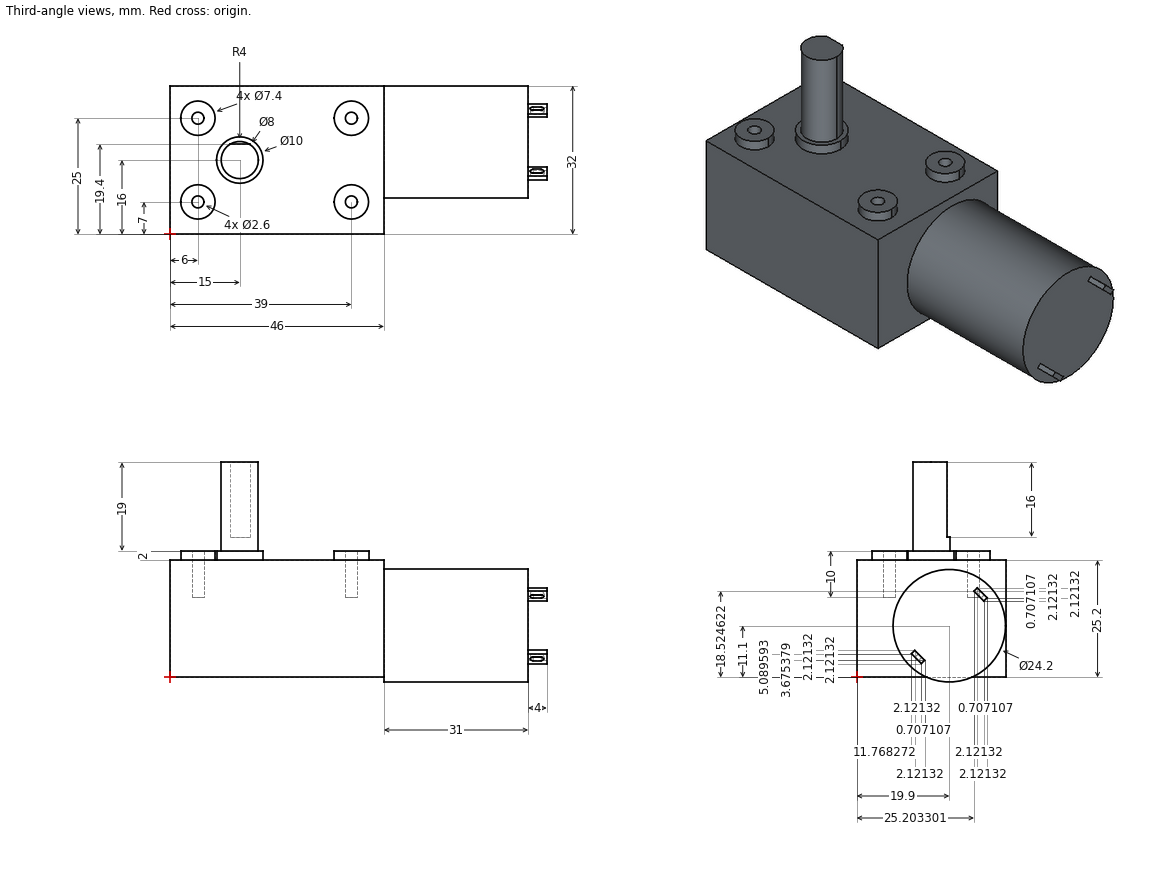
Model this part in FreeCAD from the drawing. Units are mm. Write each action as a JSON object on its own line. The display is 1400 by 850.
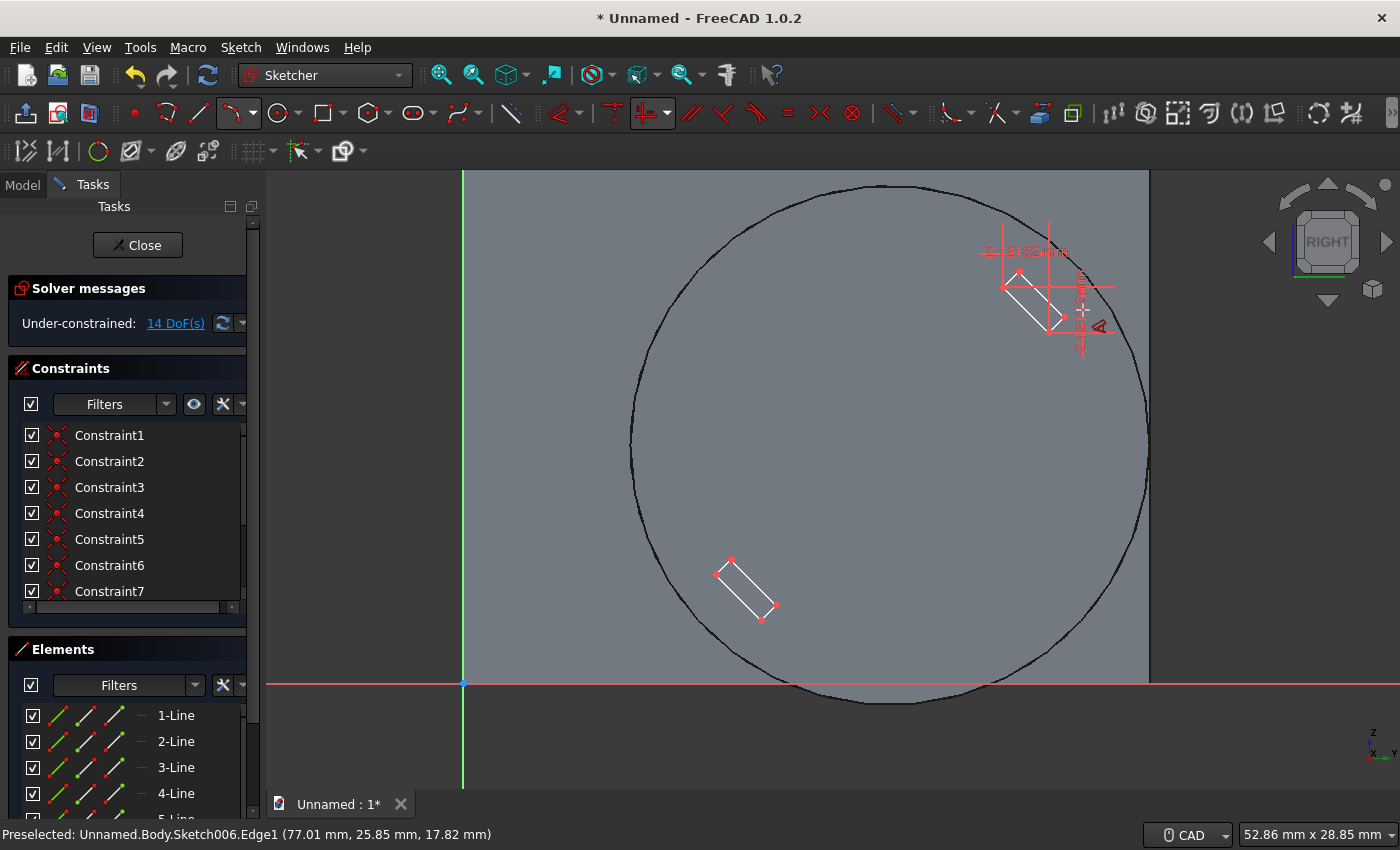
{"action": "left_click", "coordinate": [1050, 304]}
{"action": "left_click", "coordinate": [1041, 352]}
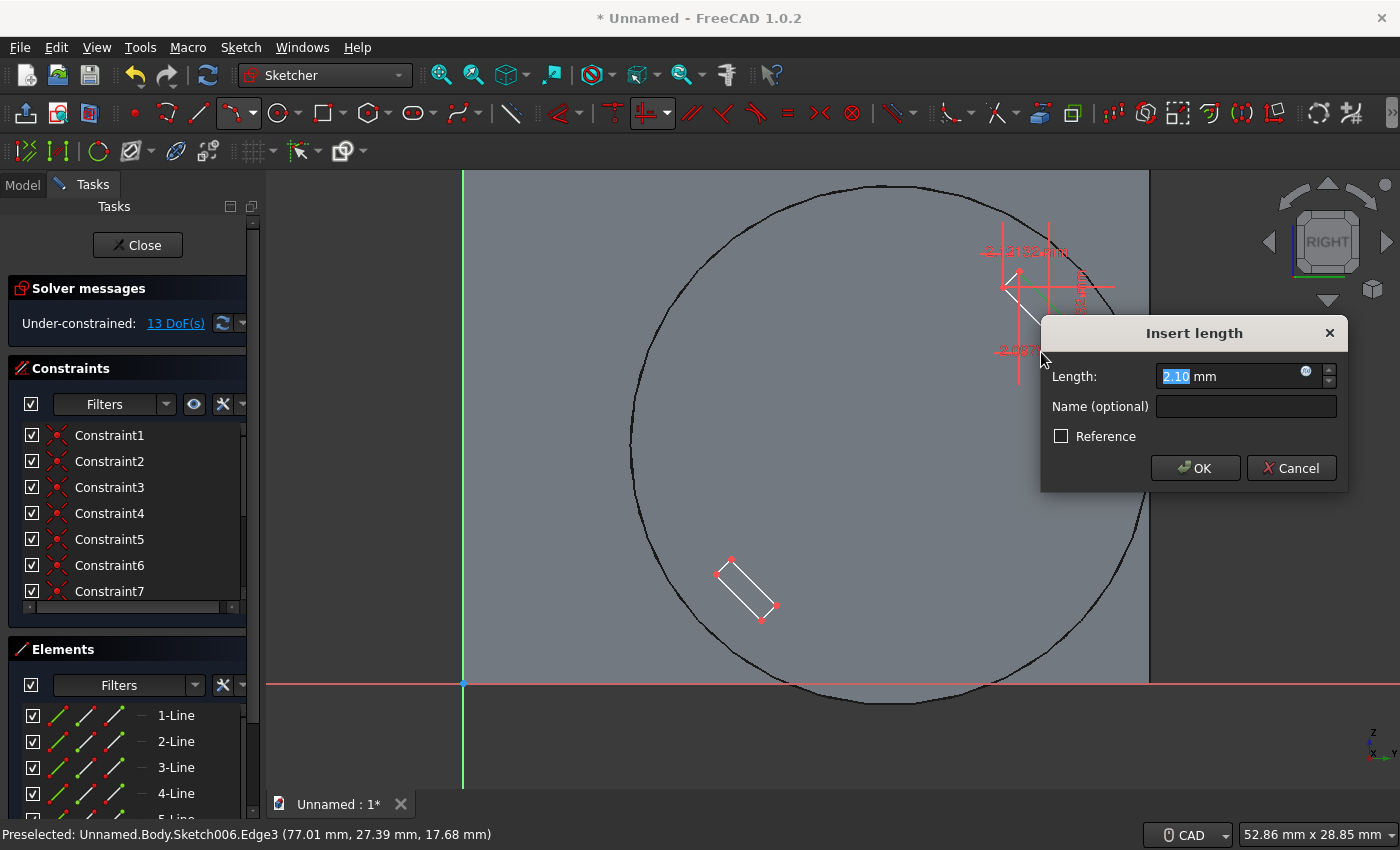
{"action": "type", "text": "2.12132"}
{"action": "key", "text": "Return"}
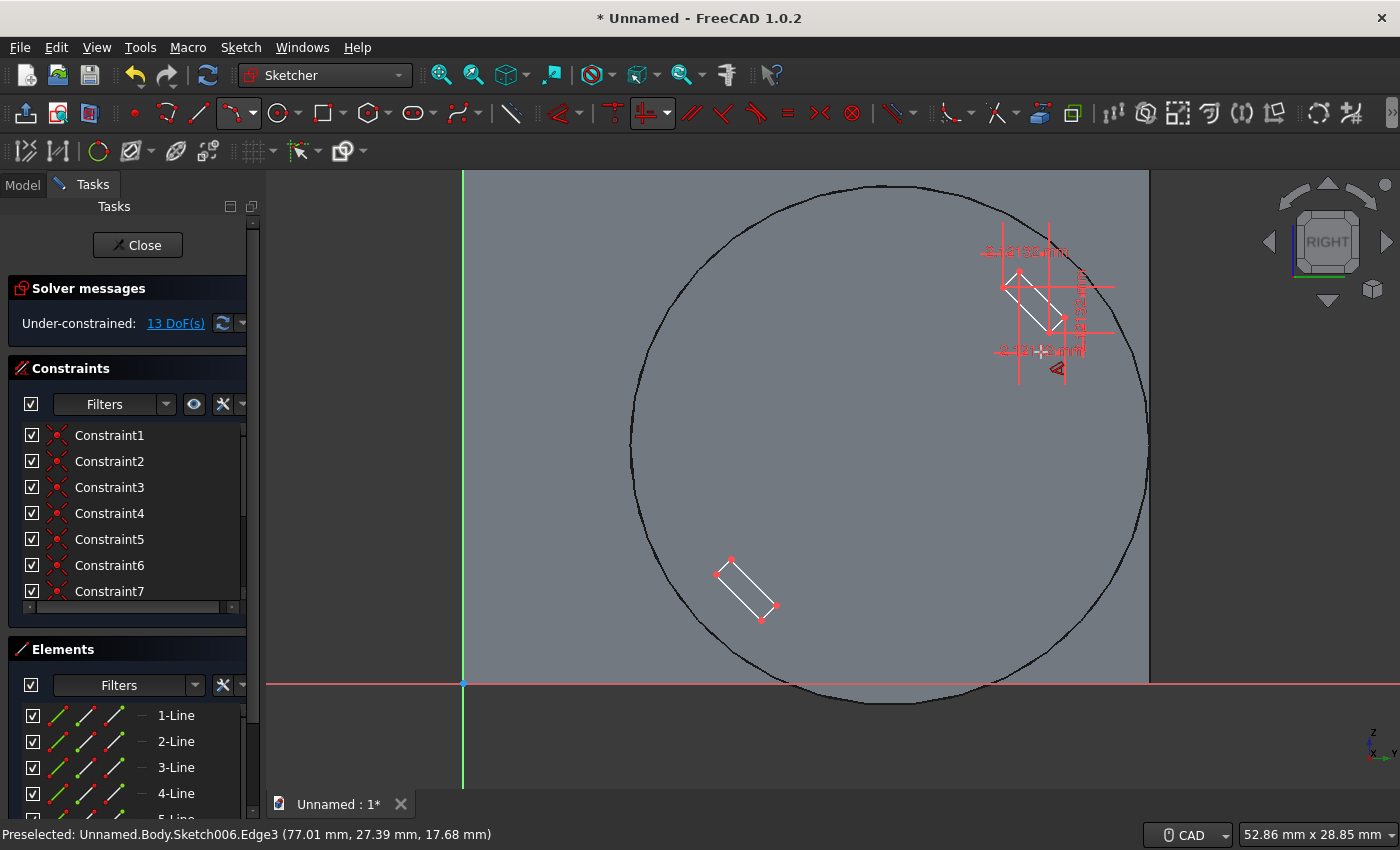
{"action": "left_click", "coordinate": [1051, 304]}
{"action": "left_click", "coordinate": [1099, 284]}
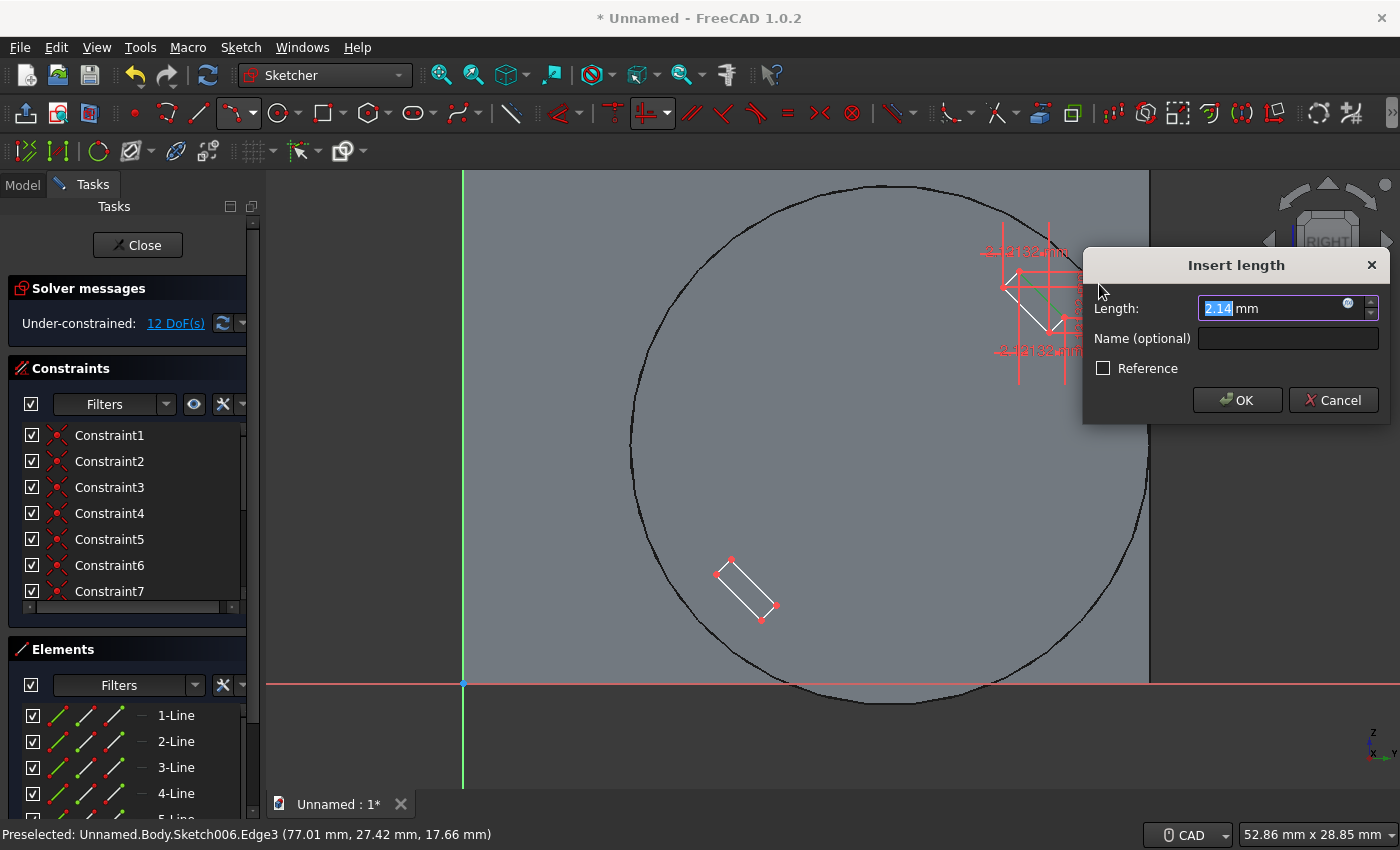
{"action": "type", "text": "2.12132"}
{"action": "key", "text": "Return"}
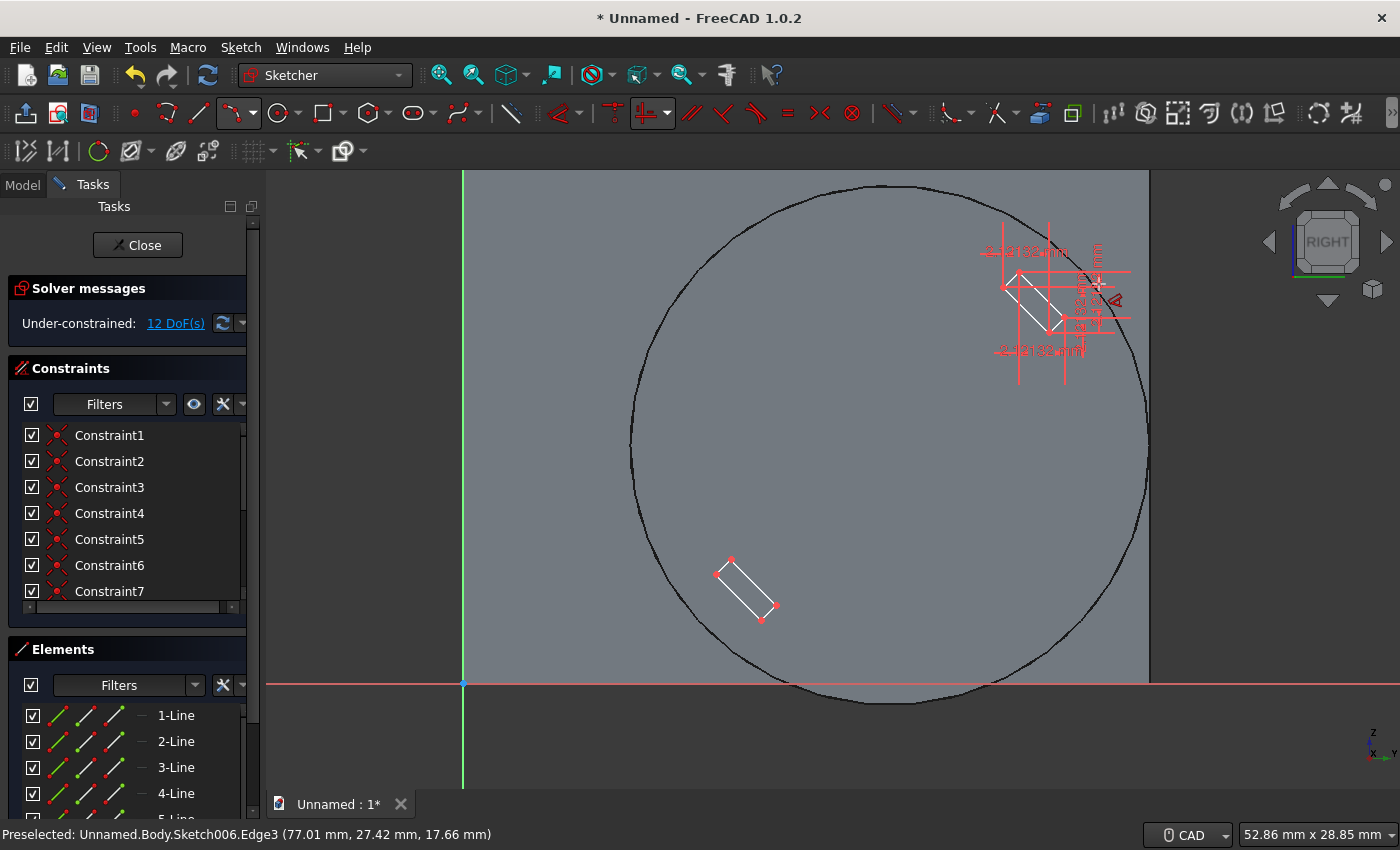
{"action": "left_click", "coordinate": [730, 589]}
{"action": "left_click", "coordinate": [739, 655]}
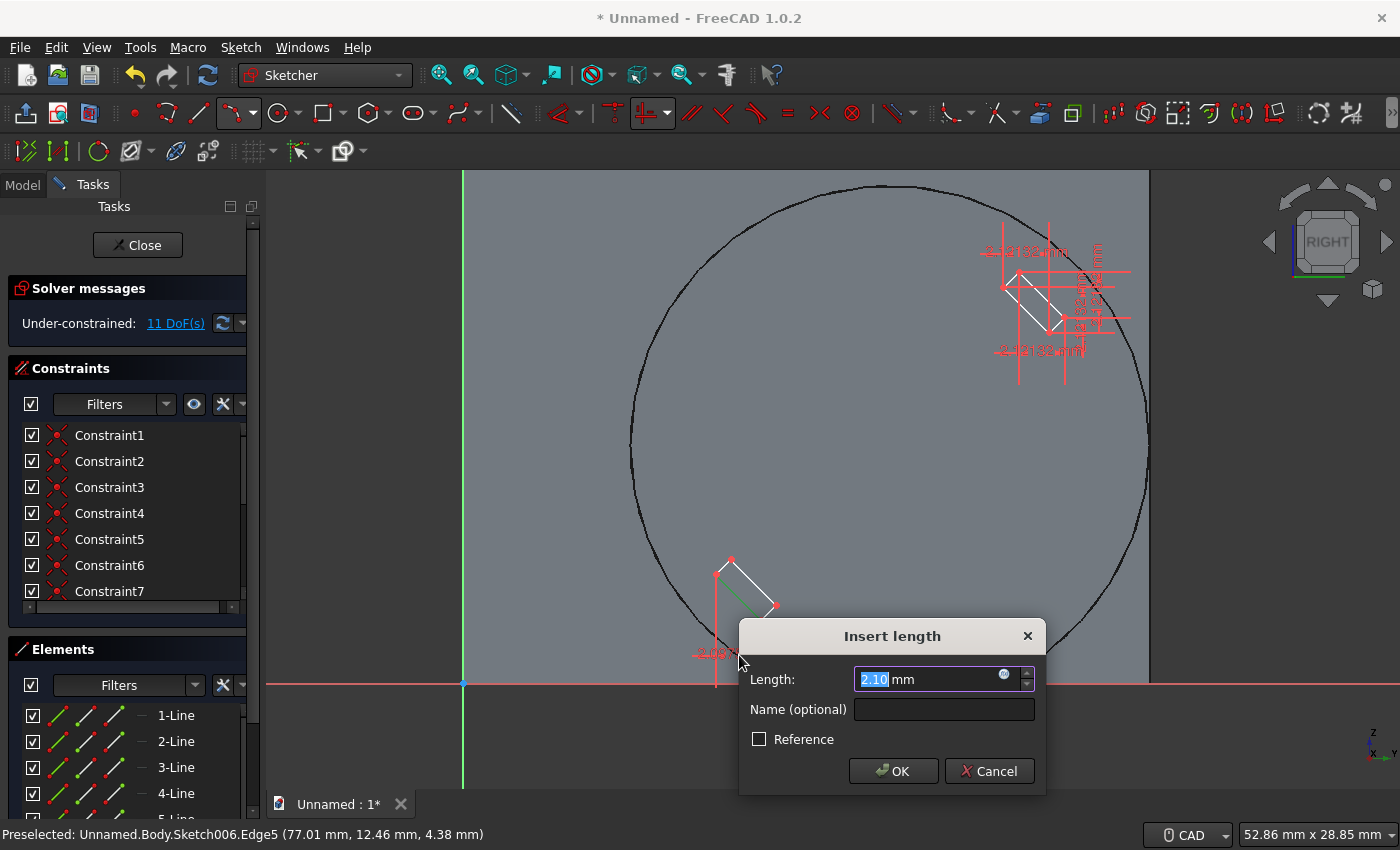
{"action": "type", "text": "2.12132"}
{"action": "key", "text": "Return"}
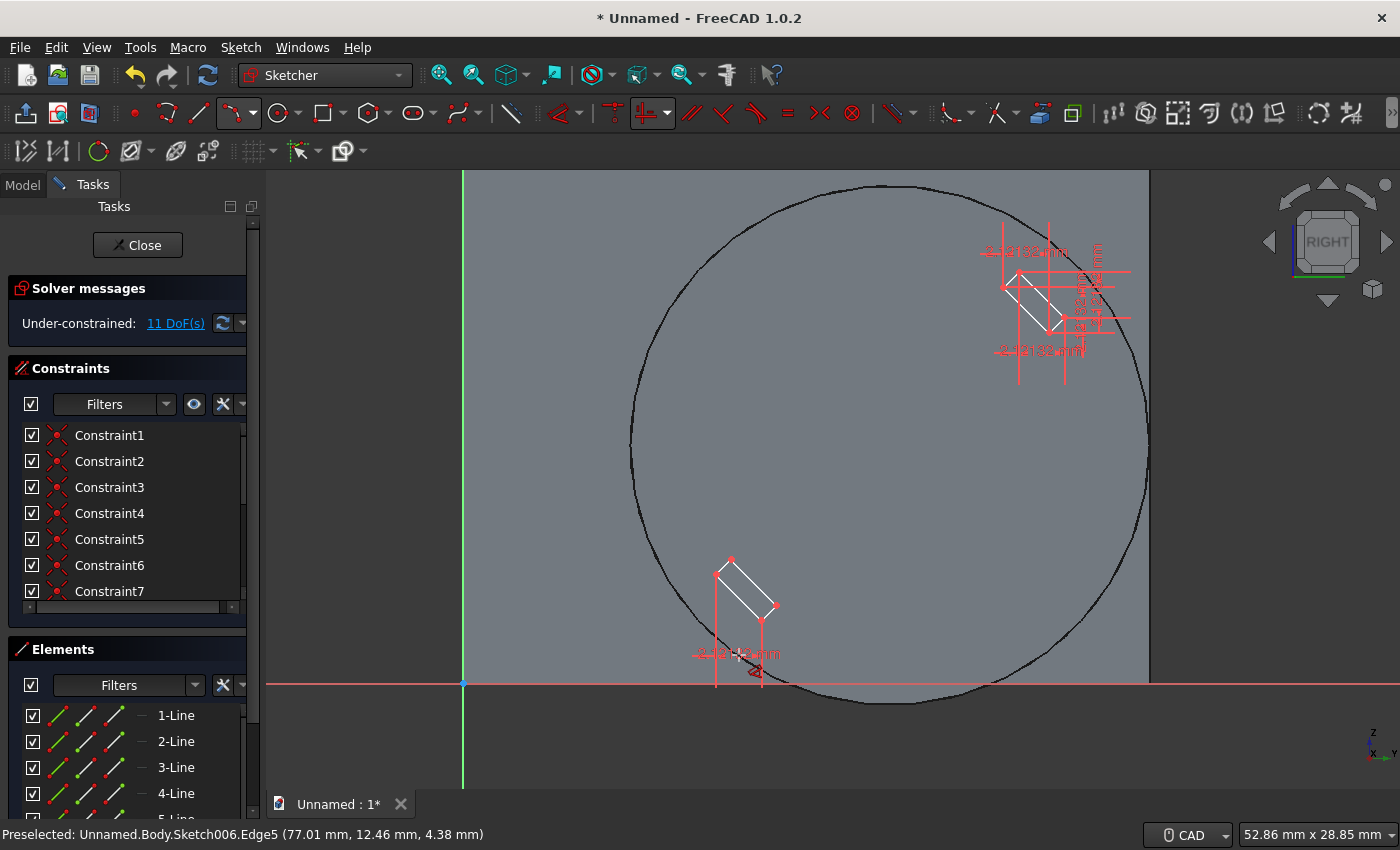
{"action": "left_click", "coordinate": [730, 589]}
{"action": "left_click", "coordinate": [682, 598]}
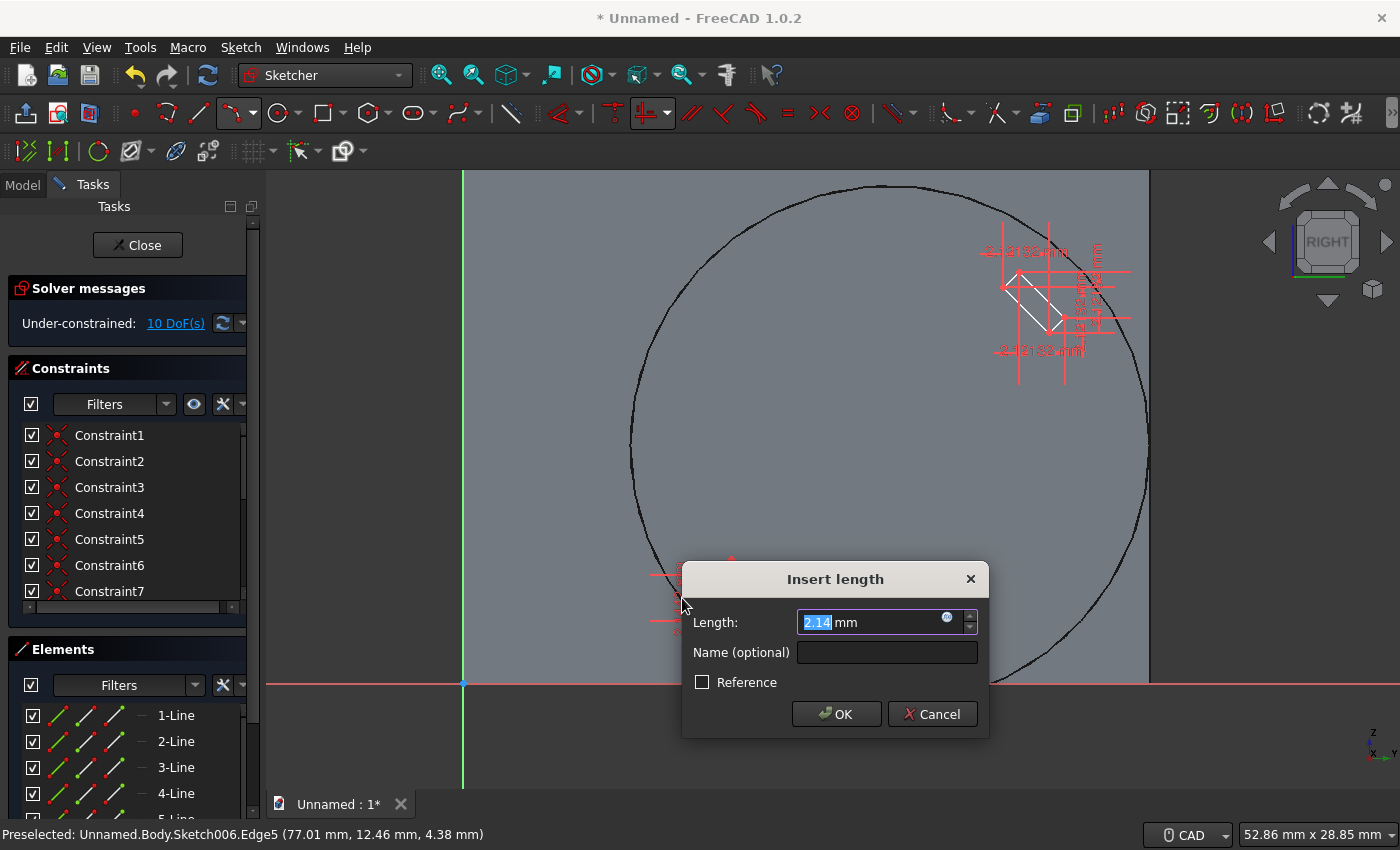
{"action": "type", "text": "2.12132"}
{"action": "key", "text": "Return"}